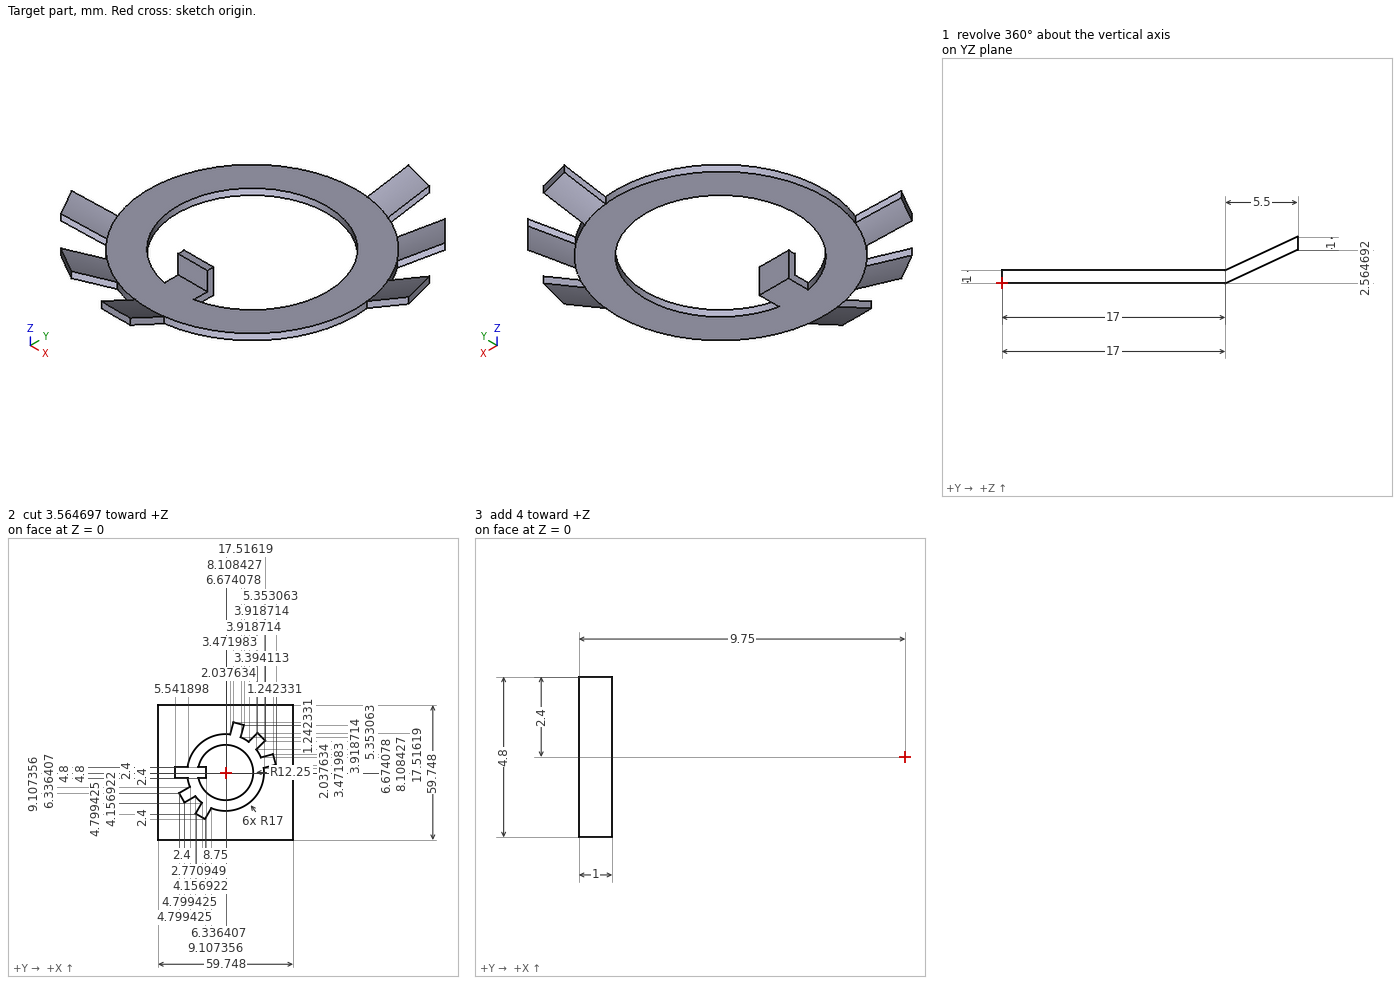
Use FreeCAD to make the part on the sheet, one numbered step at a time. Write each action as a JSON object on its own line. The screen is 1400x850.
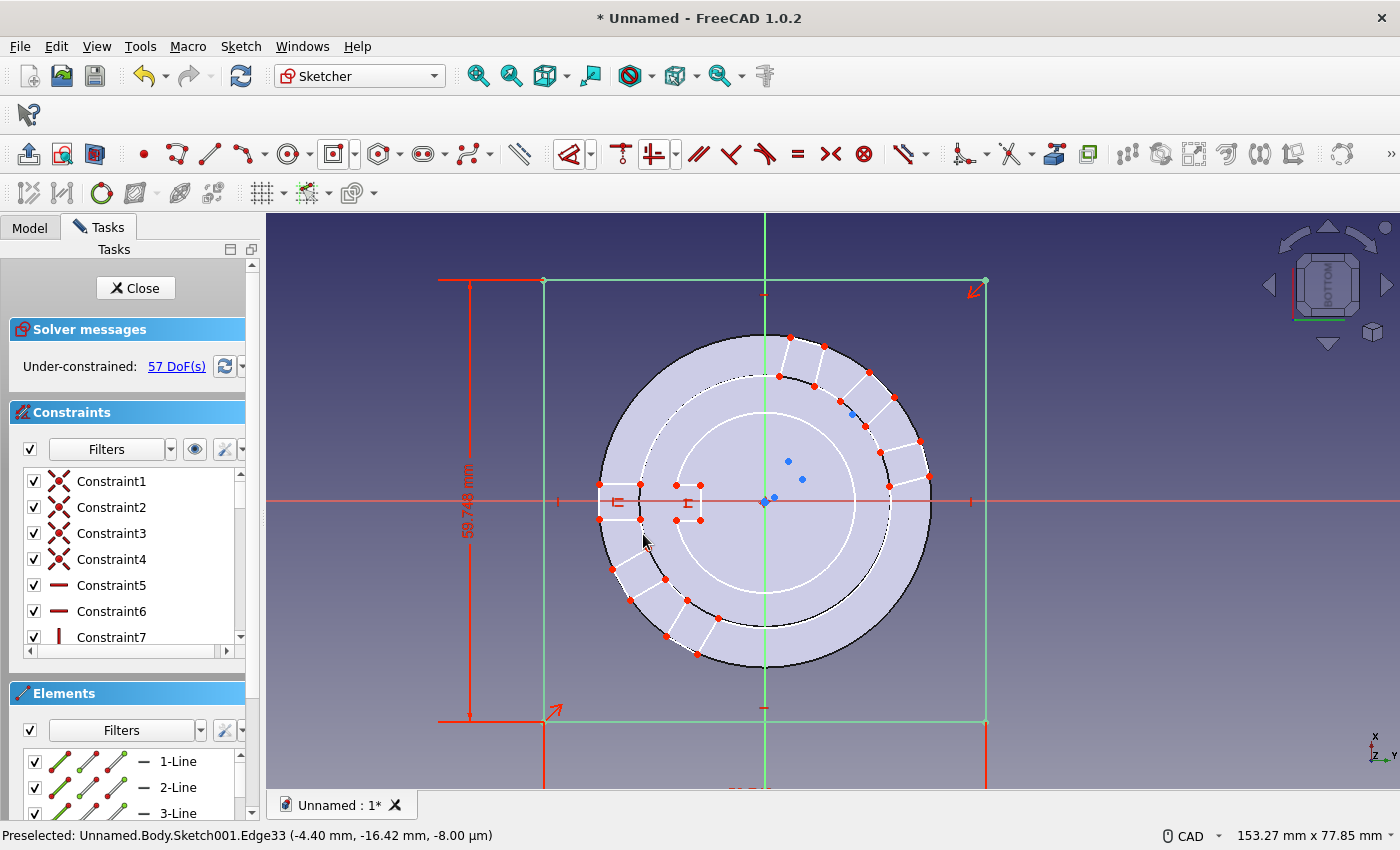
{"action": "left_click", "coordinate": [799, 586]}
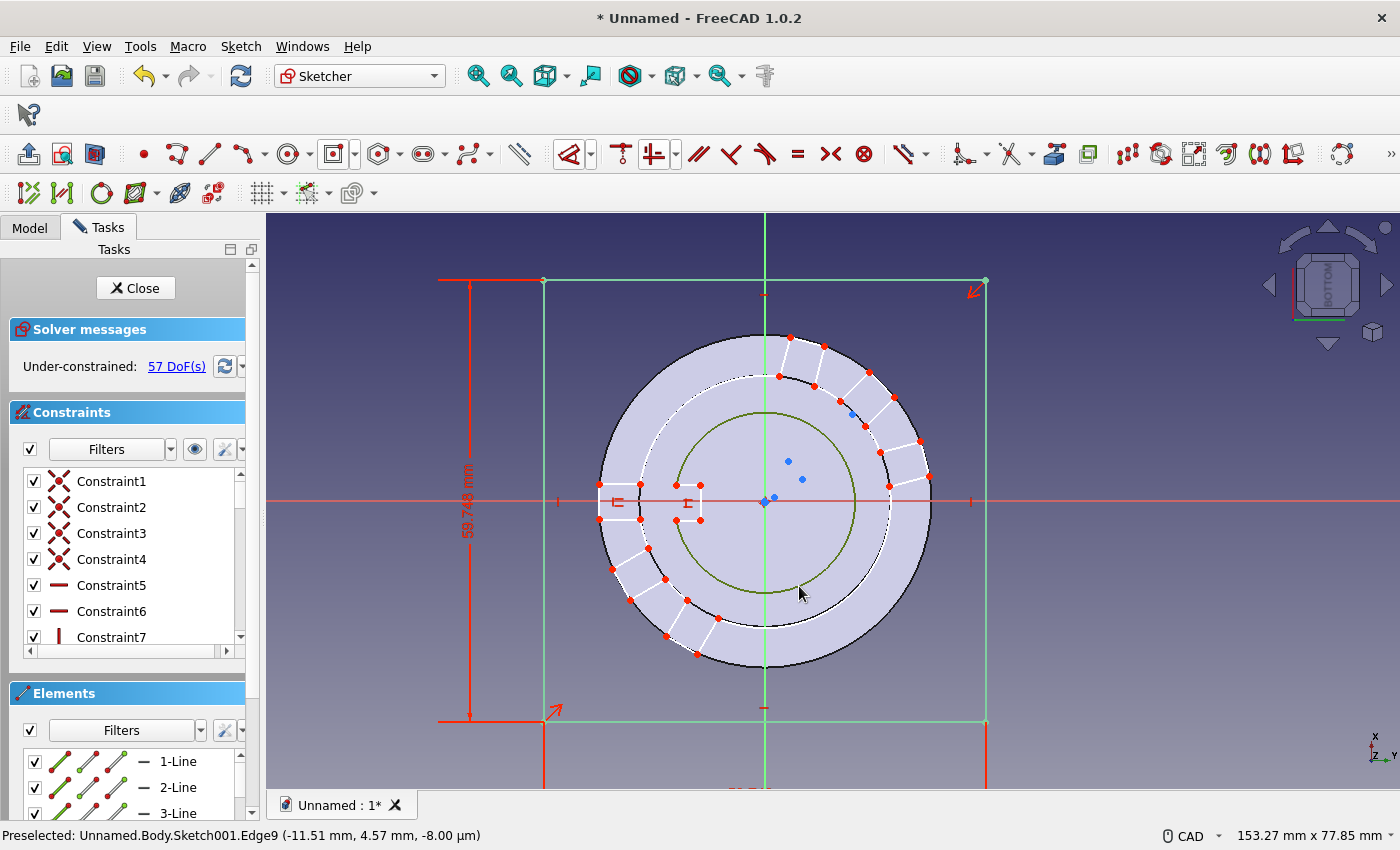
{"action": "scroll", "coordinate": [672, 586], "scroll_direction": "up", "scroll_amount": 3}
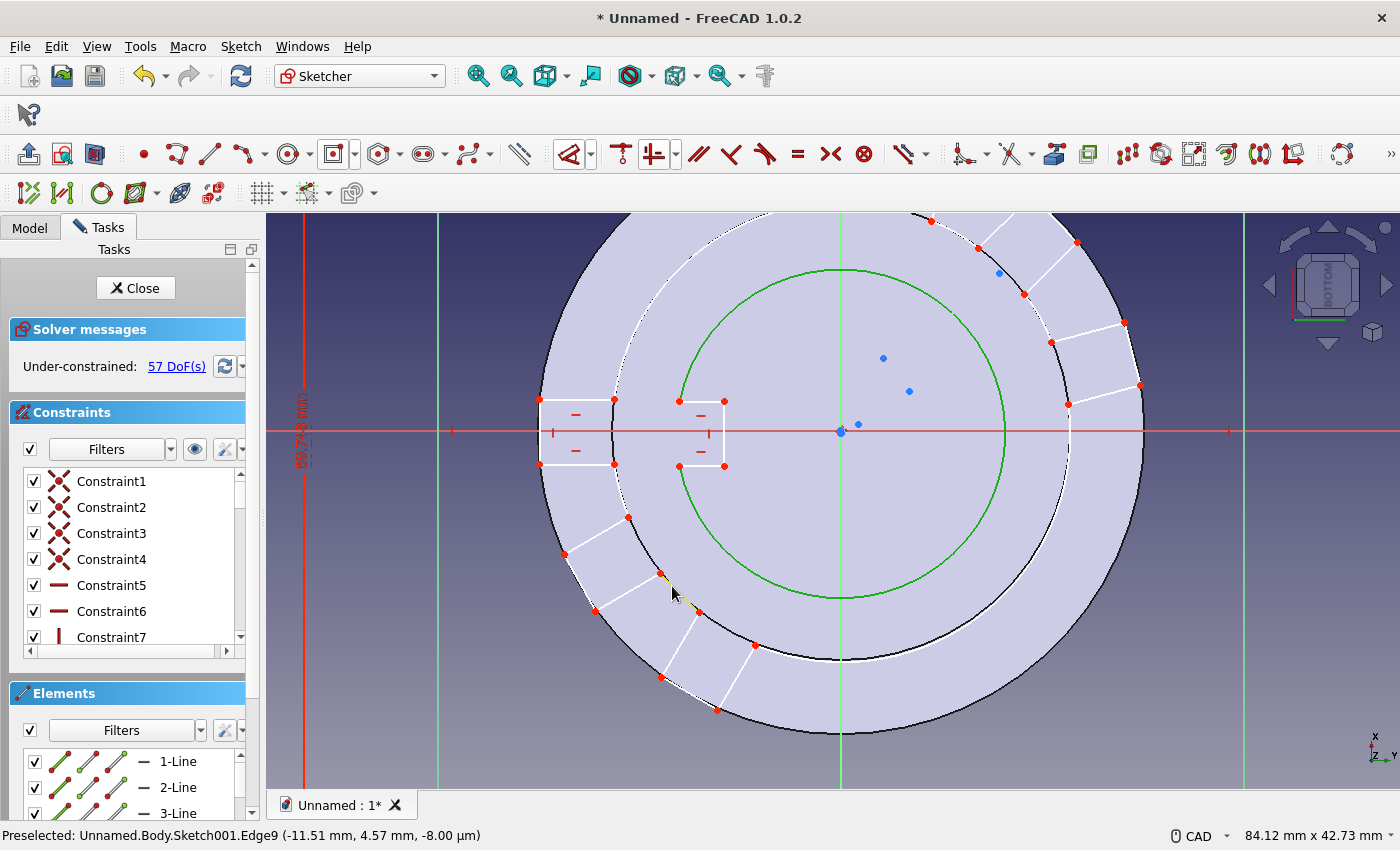
{"action": "left_click", "coordinate": [672, 586]}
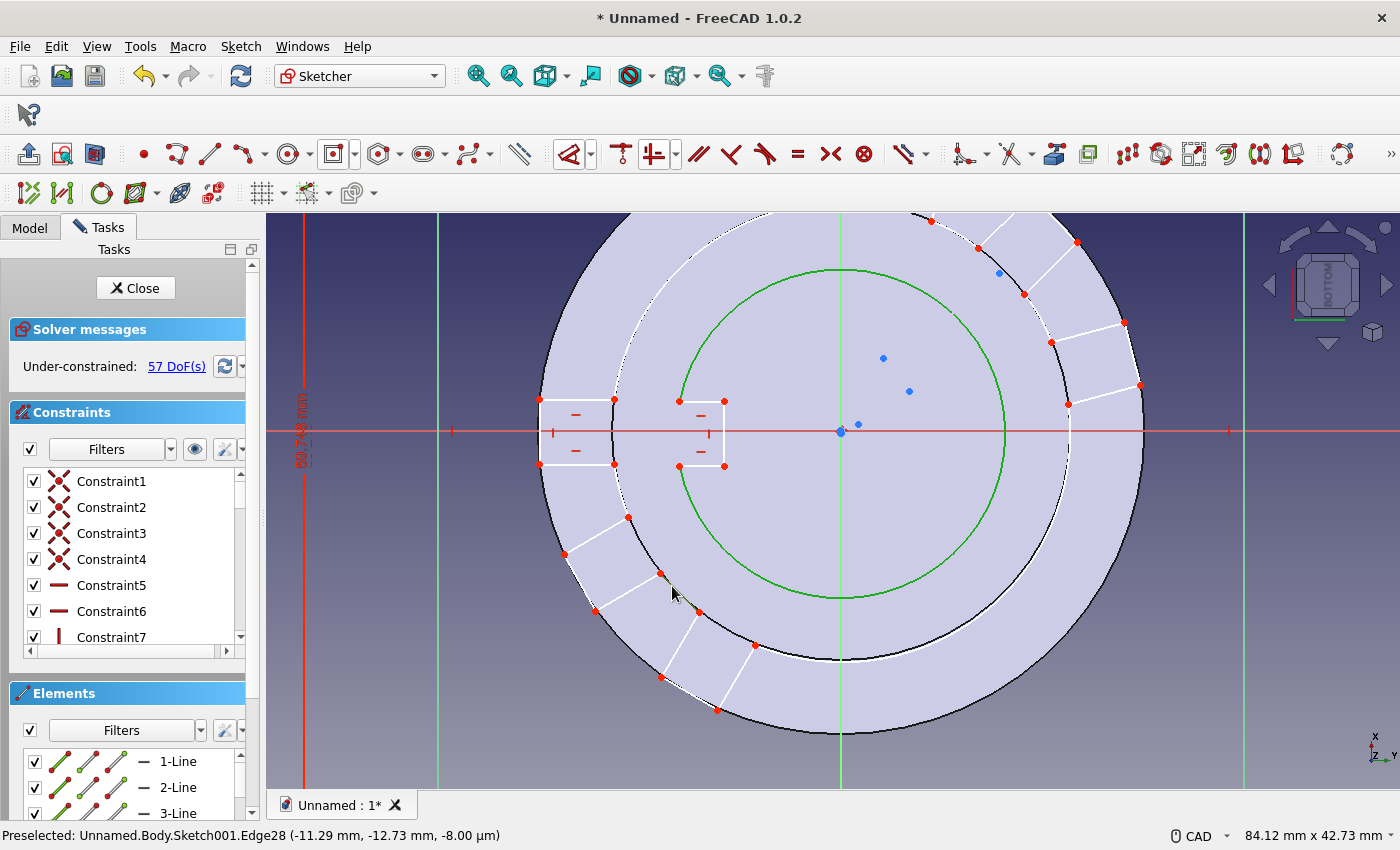
{"action": "key", "text": "c"}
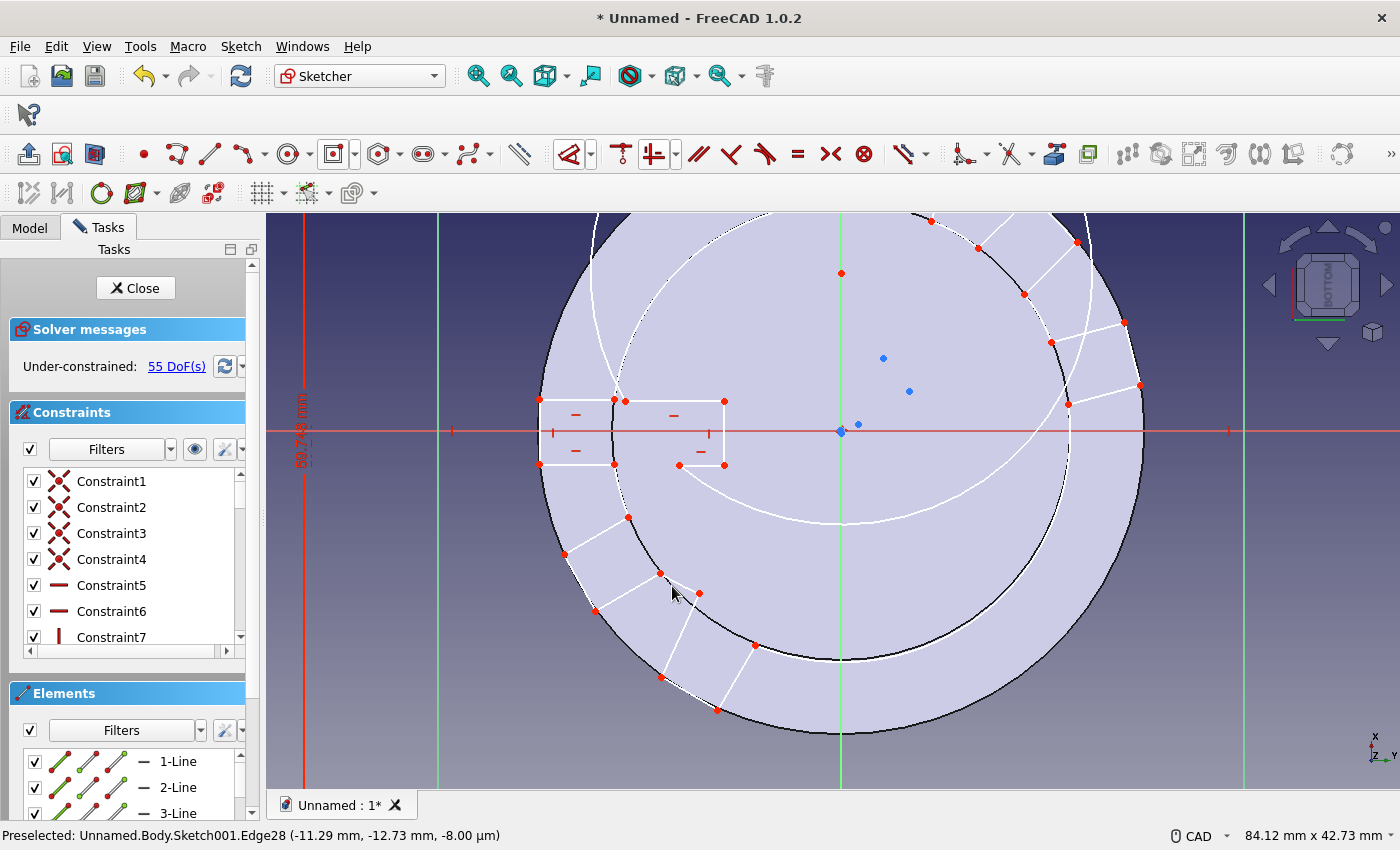
{"action": "left_click", "coordinate": [1063, 391]}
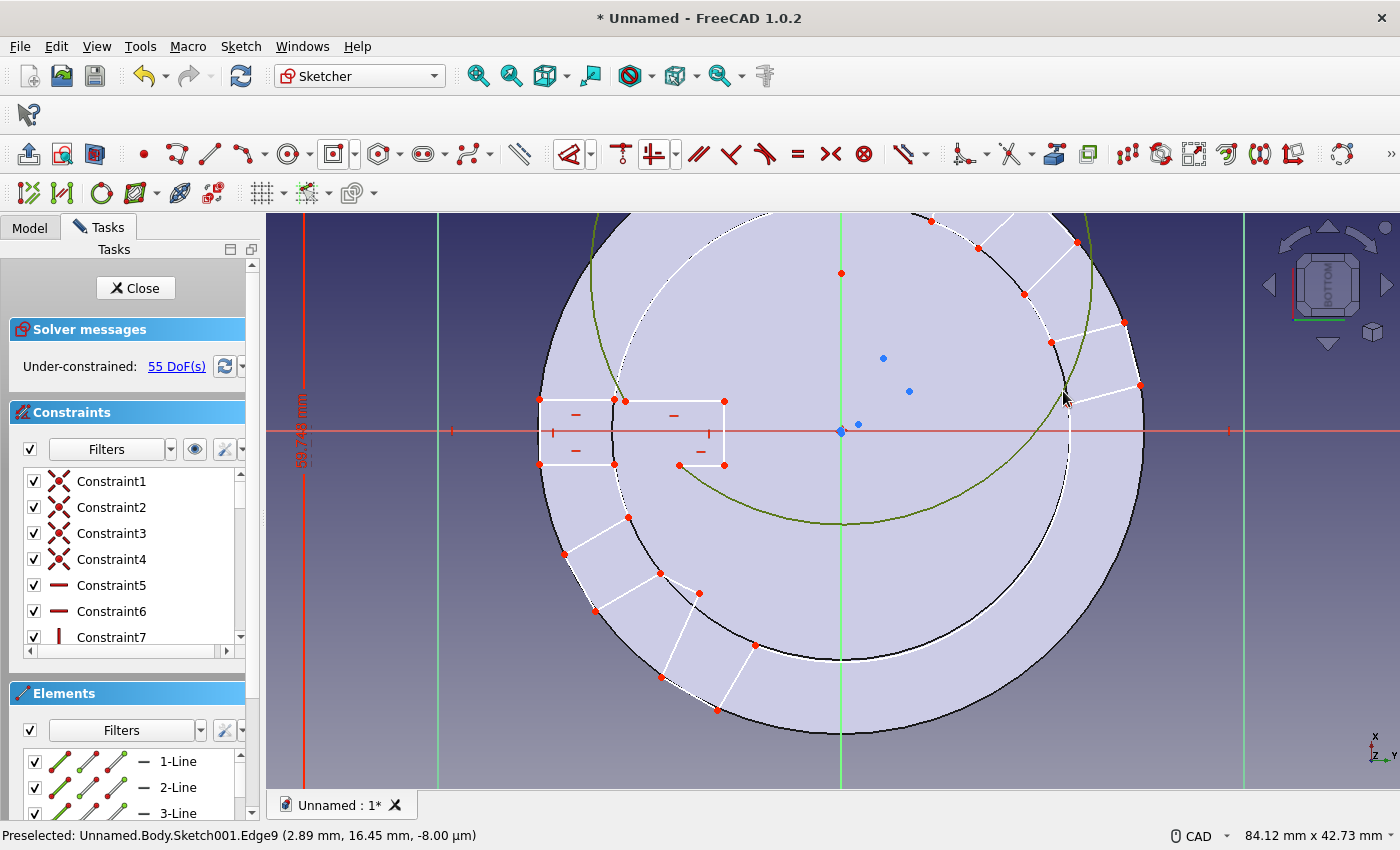
{"action": "left_click", "coordinate": [896, 656]}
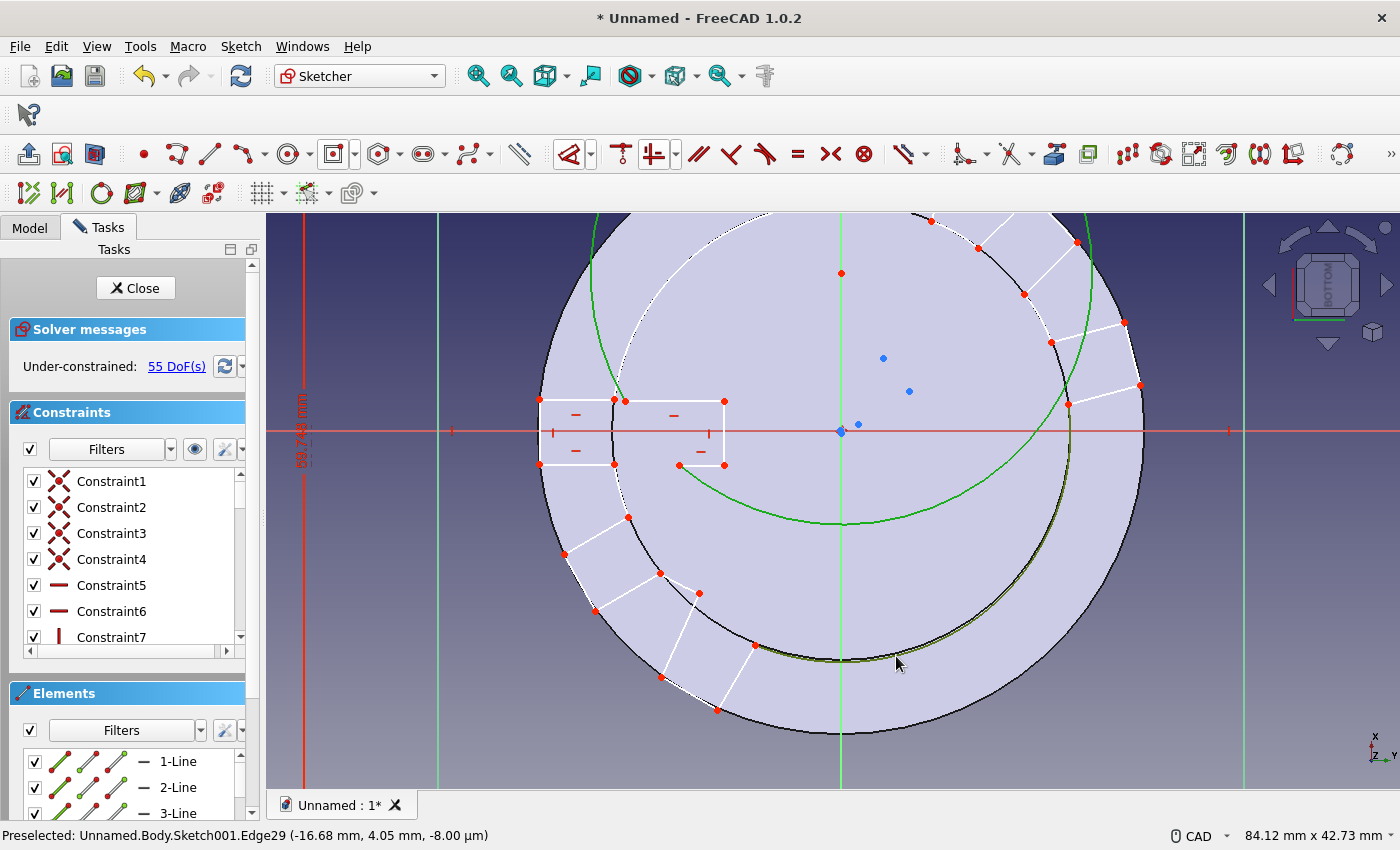
{"action": "left_click", "coordinate": [621, 154]}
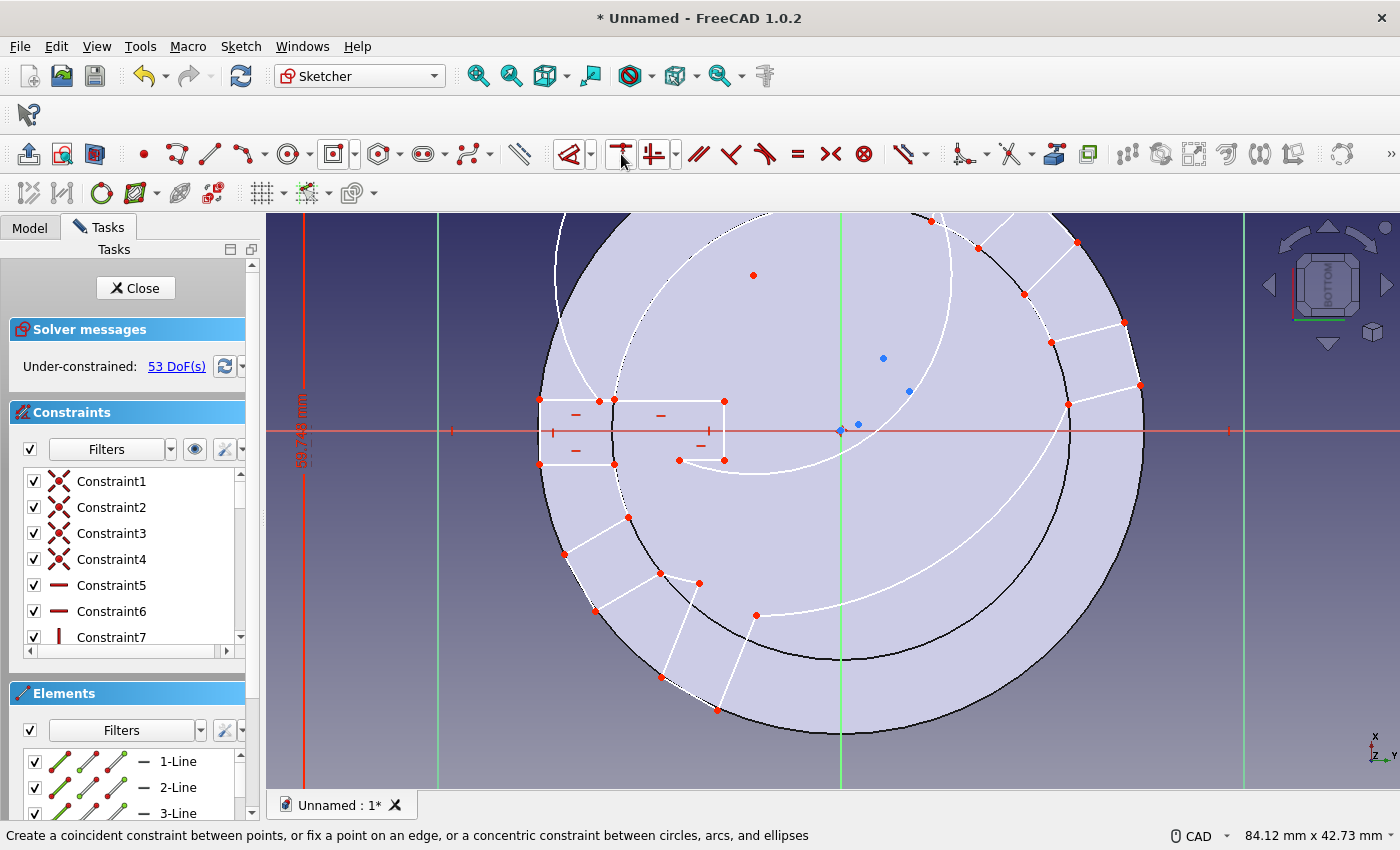
{"action": "left_click", "coordinate": [947, 319]}